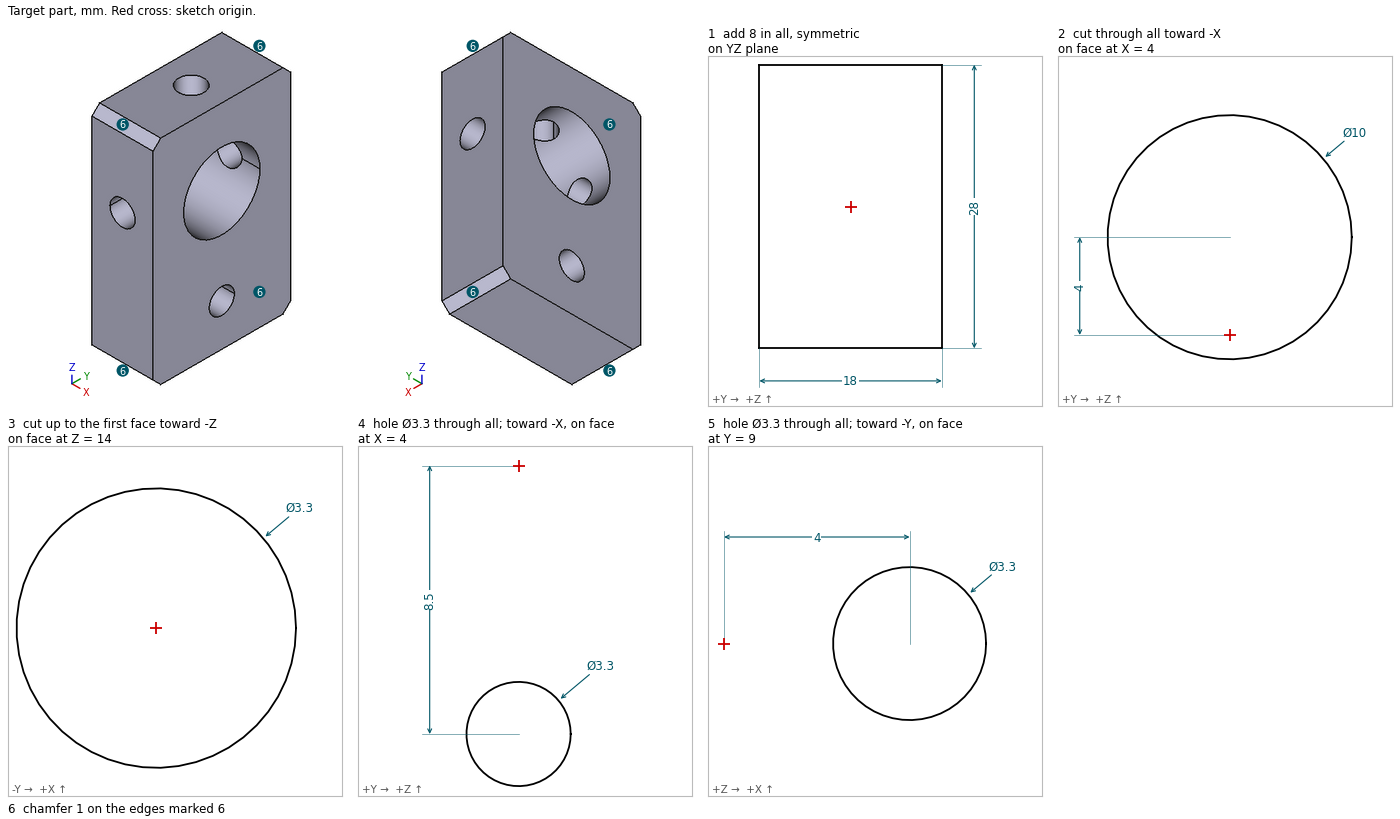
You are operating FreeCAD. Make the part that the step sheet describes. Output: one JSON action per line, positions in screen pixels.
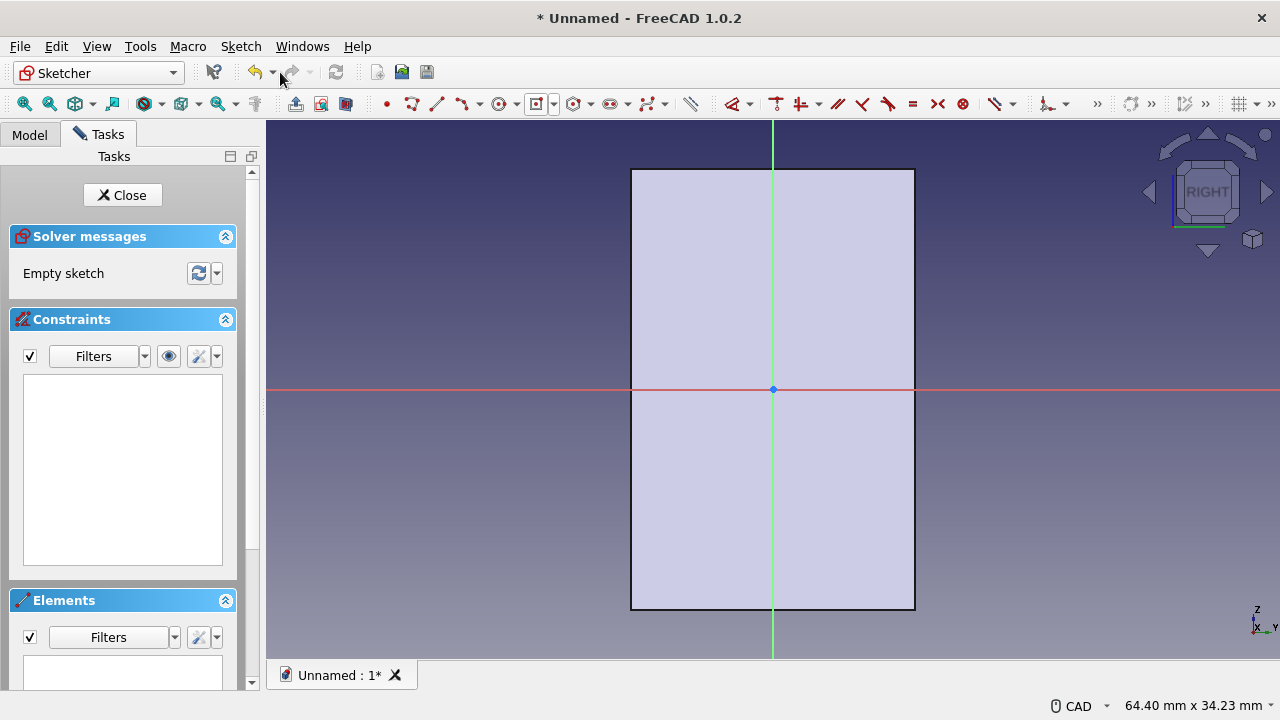
{"action": "scroll", "coordinate": [829, 275], "scroll_direction": "up", "scroll_amount": 4}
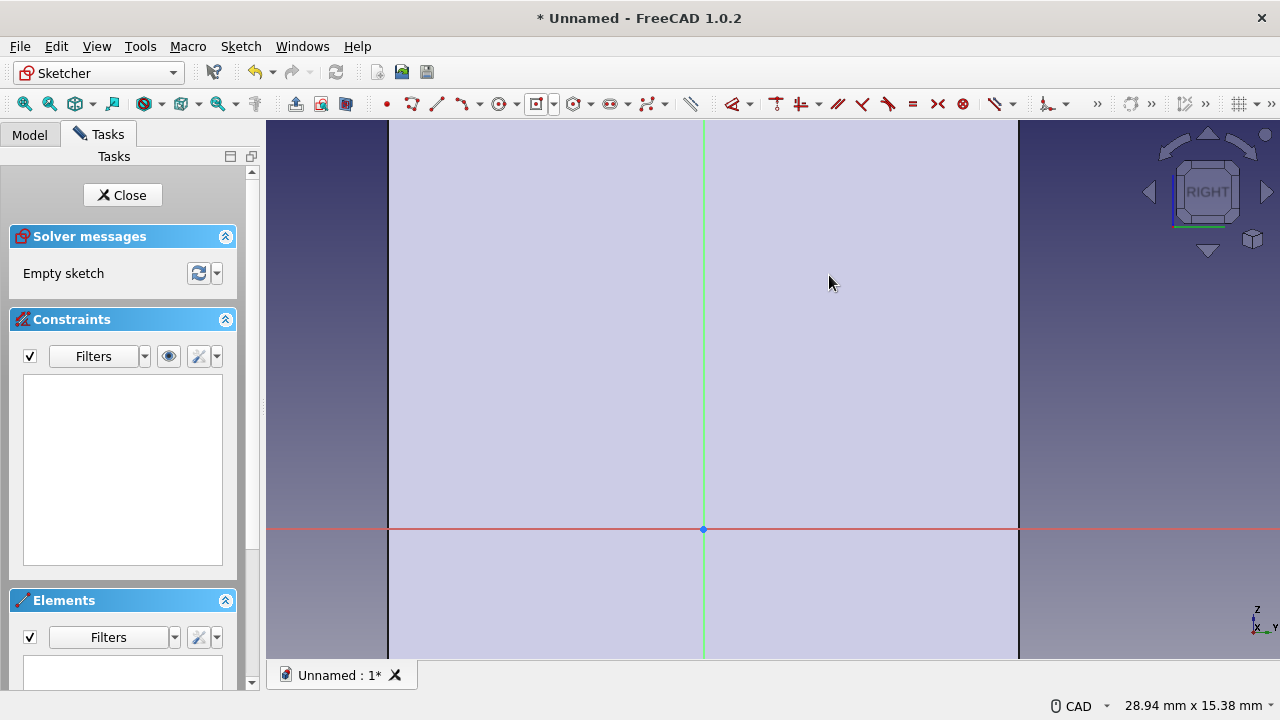
{"action": "left_click", "coordinate": [498, 104]}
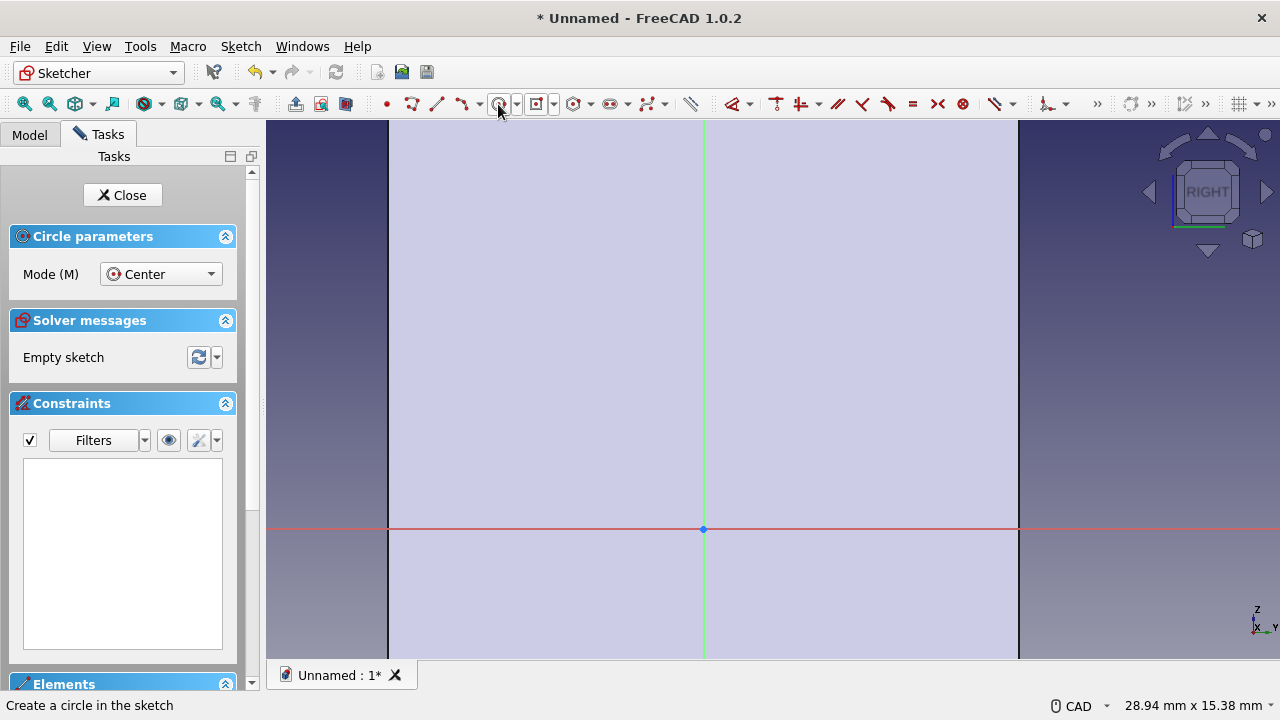
{"action": "left_click", "coordinate": [704, 389]}
{"action": "left_click", "coordinate": [828, 265]}
{"action": "key", "text": "Escape"}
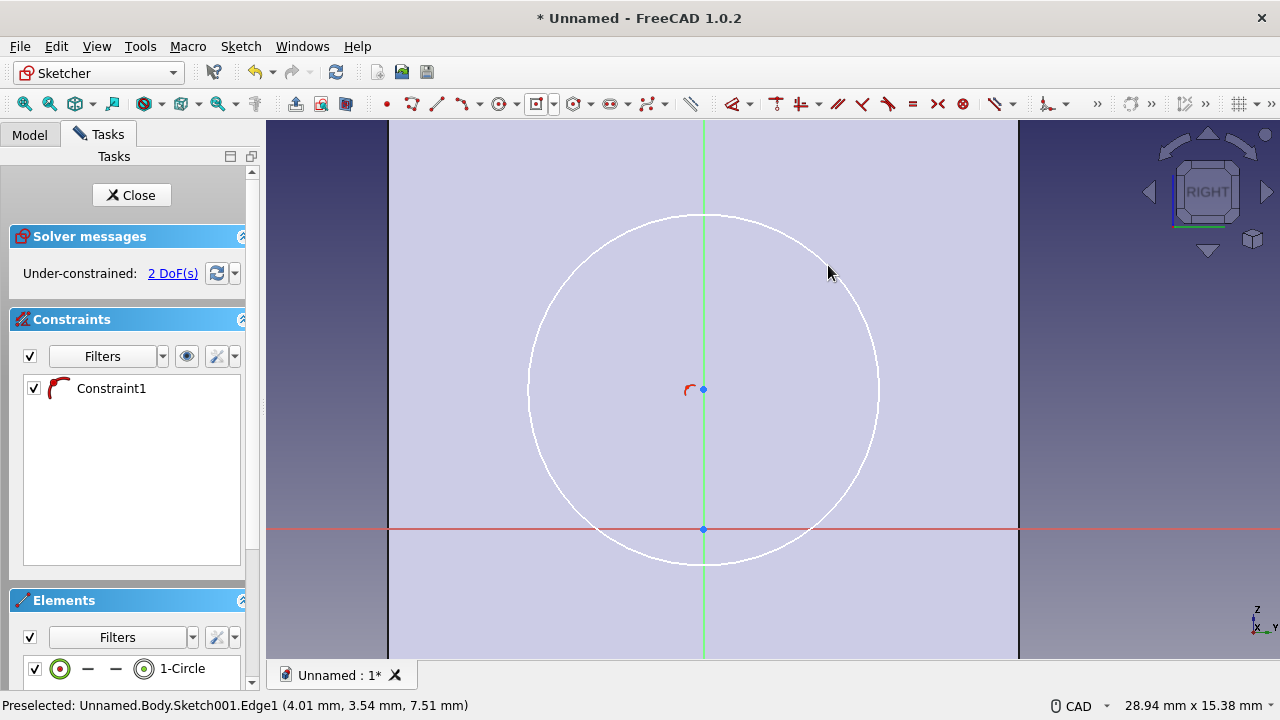
{"action": "left_click", "coordinate": [827, 265]}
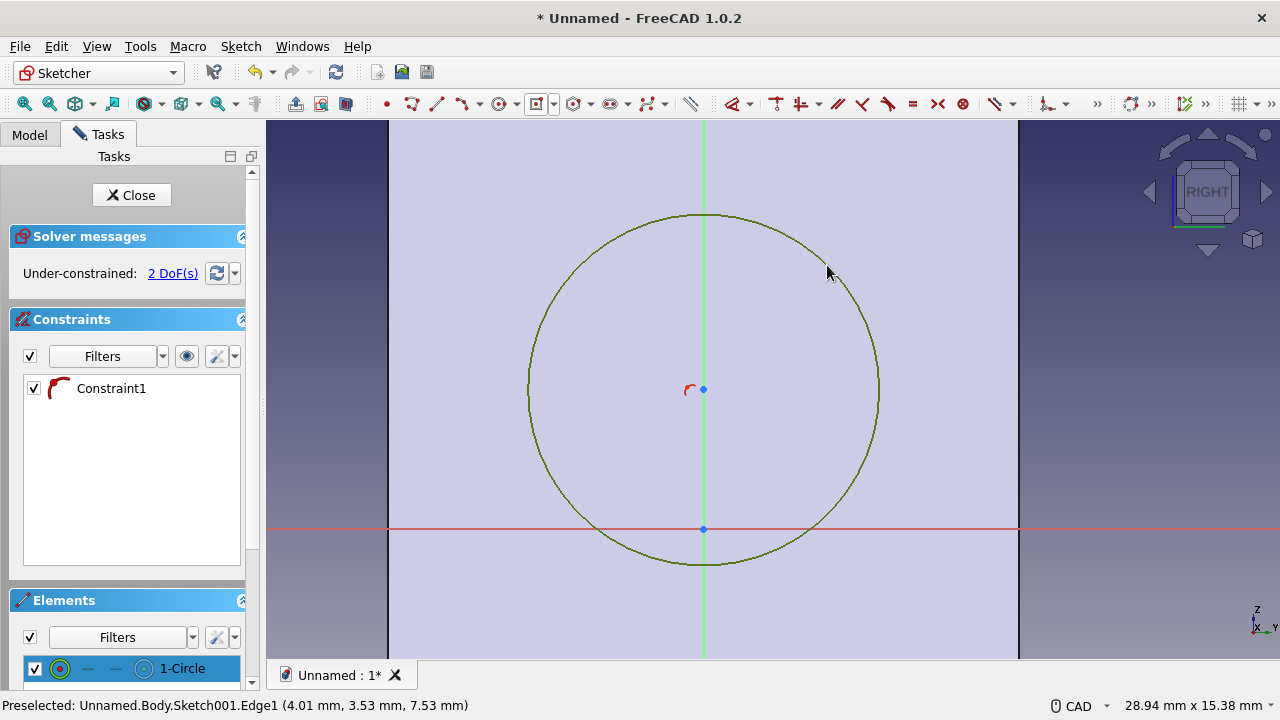
{"action": "left_click", "coordinate": [750, 104]}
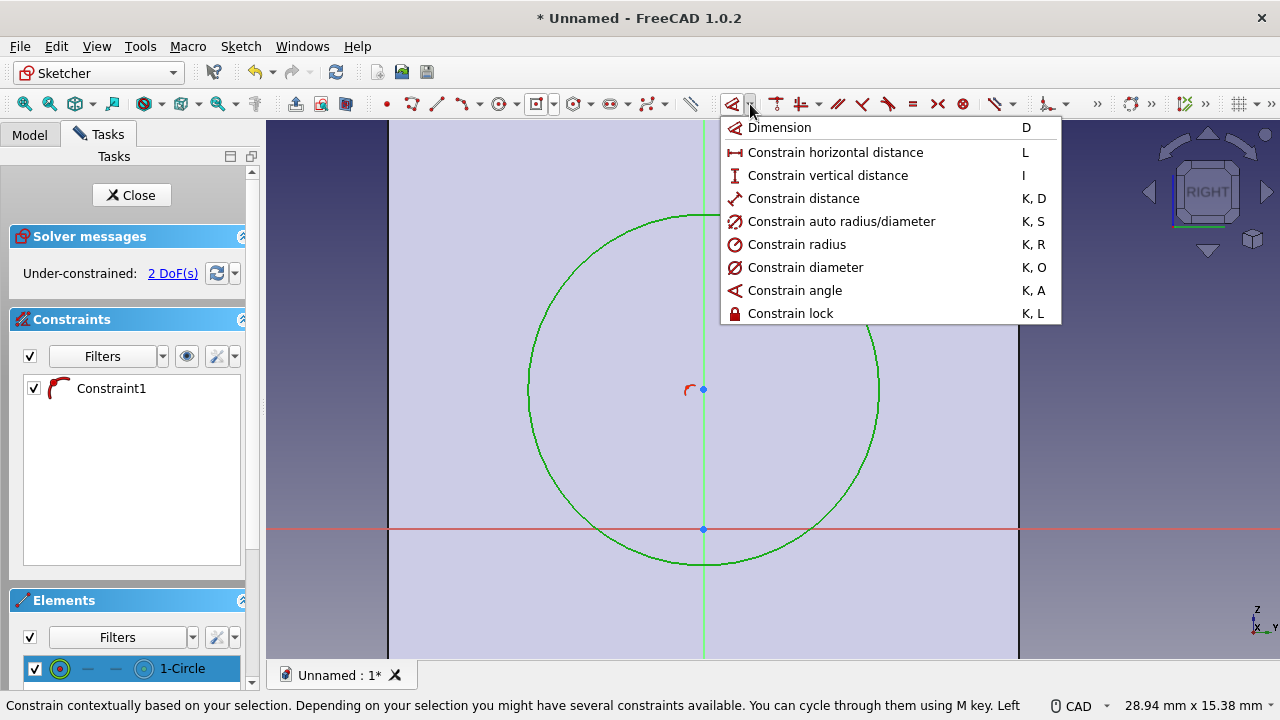
{"action": "left_click", "coordinate": [891, 268]}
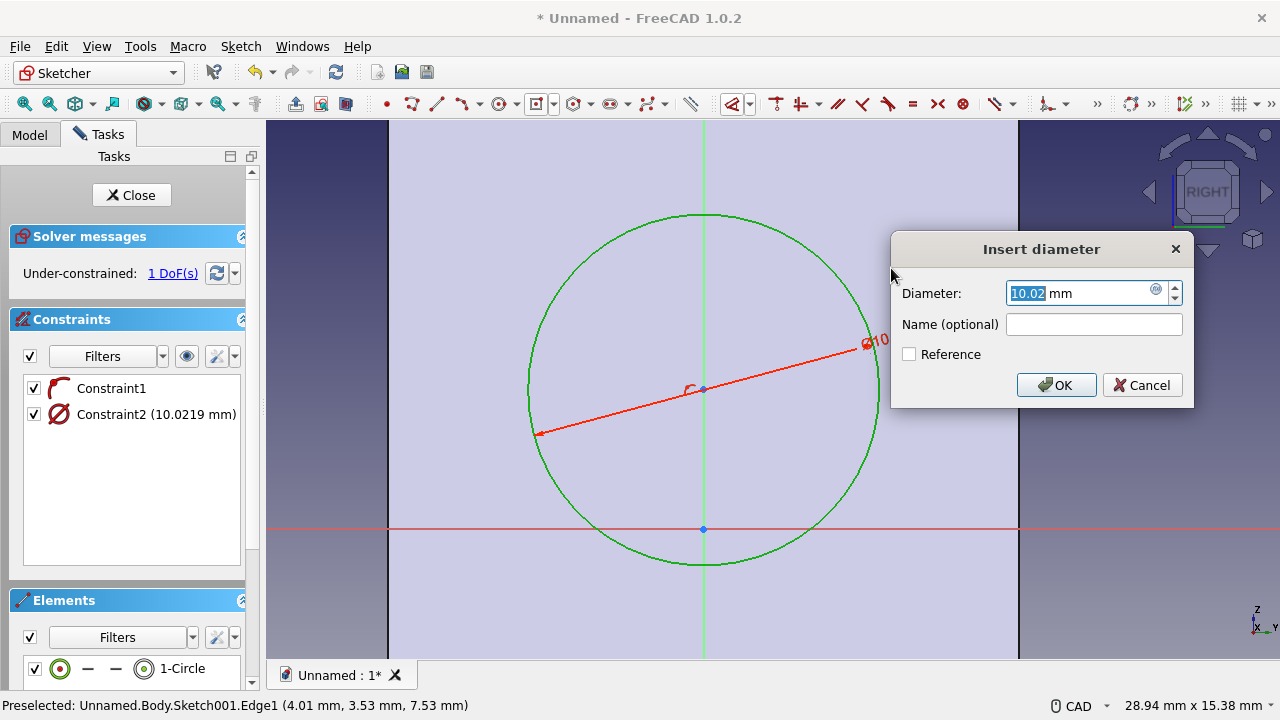
{"action": "type", "text": "10"}
{"action": "key", "text": "Return"}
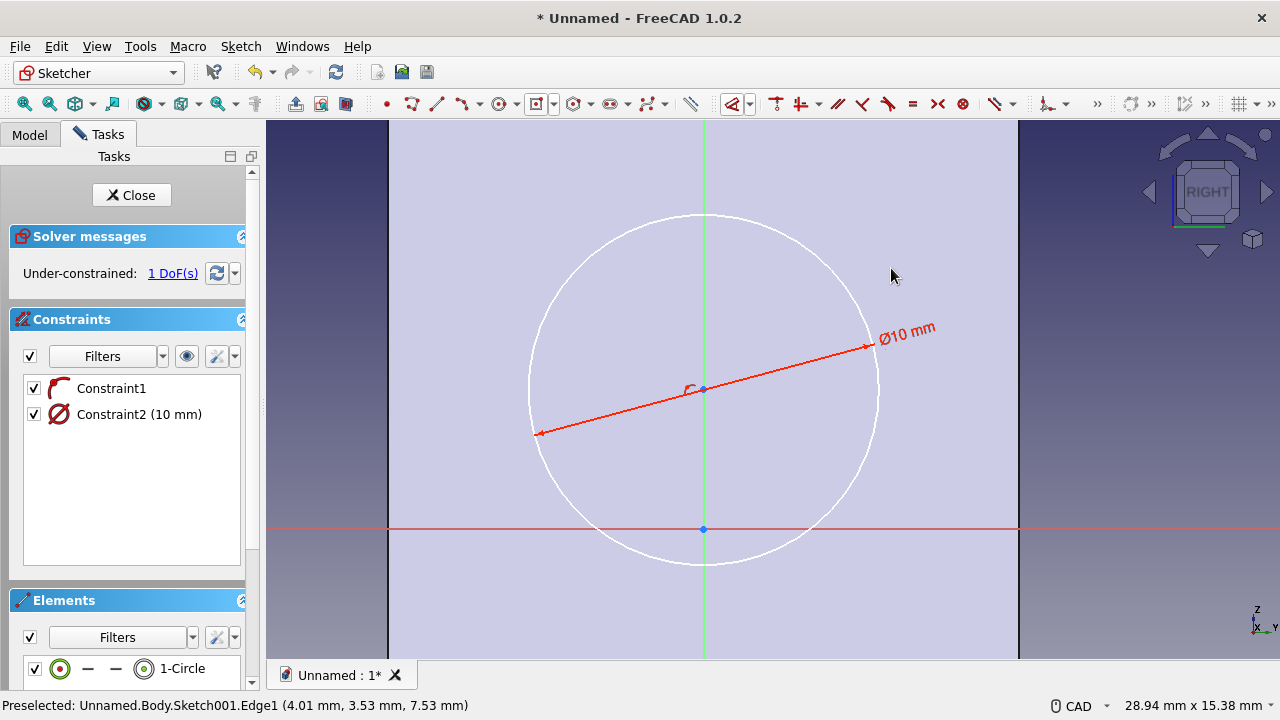
{"action": "left_click", "coordinate": [704, 390]}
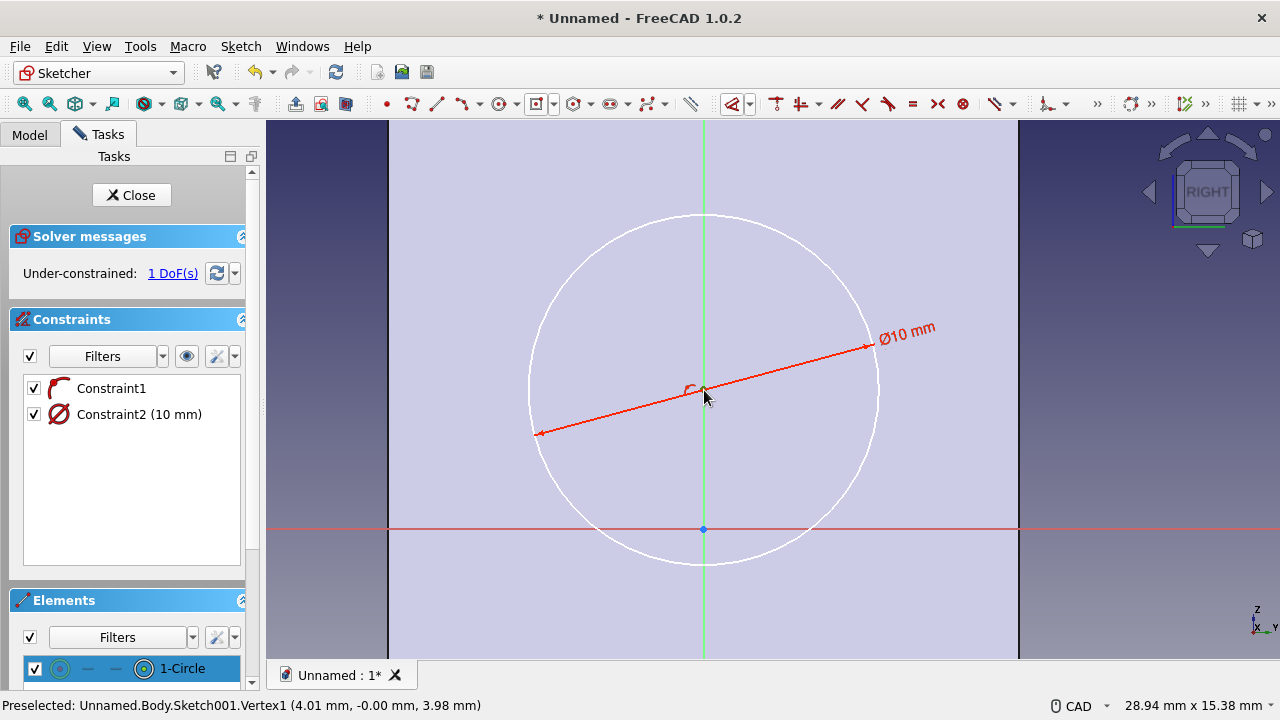
{"action": "left_click", "coordinate": [750, 104]}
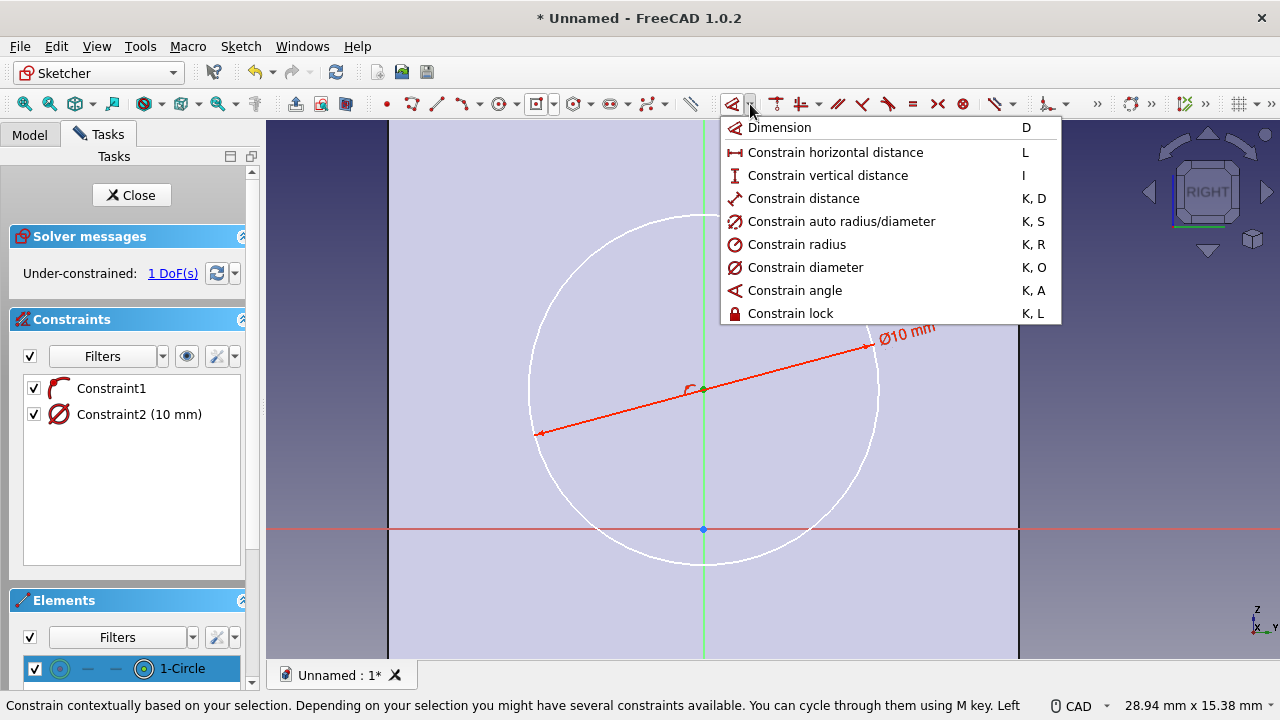
{"action": "left_click", "coordinate": [891, 176]}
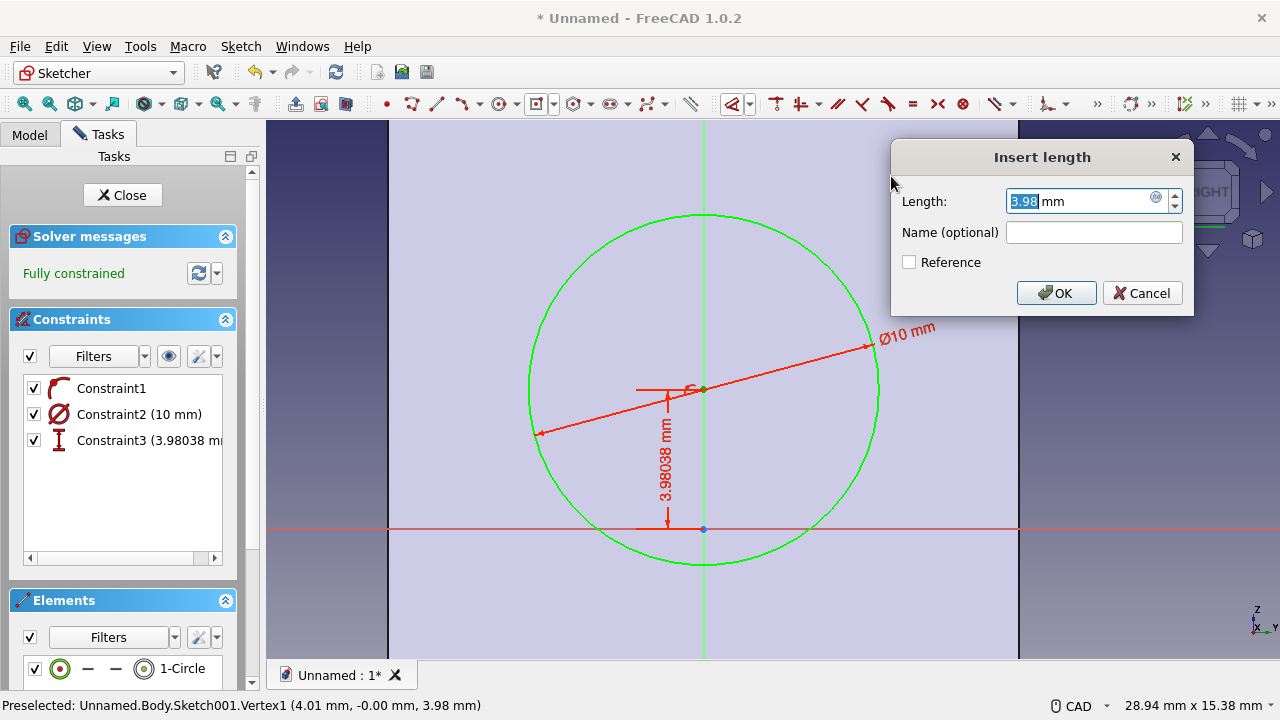
{"action": "type", "text": "4"}
{"action": "key", "text": "Return"}